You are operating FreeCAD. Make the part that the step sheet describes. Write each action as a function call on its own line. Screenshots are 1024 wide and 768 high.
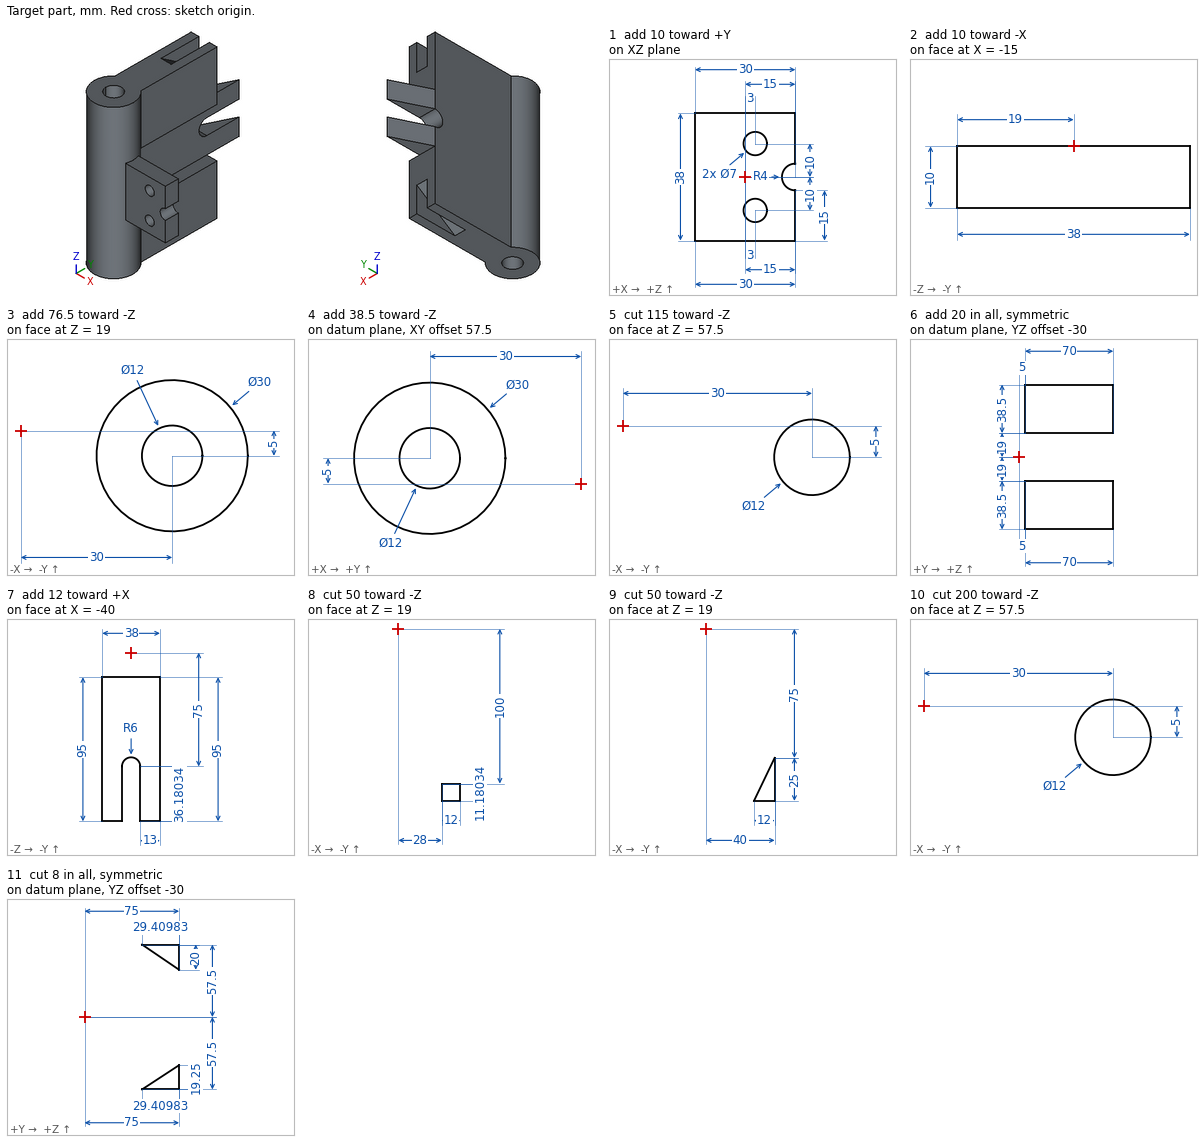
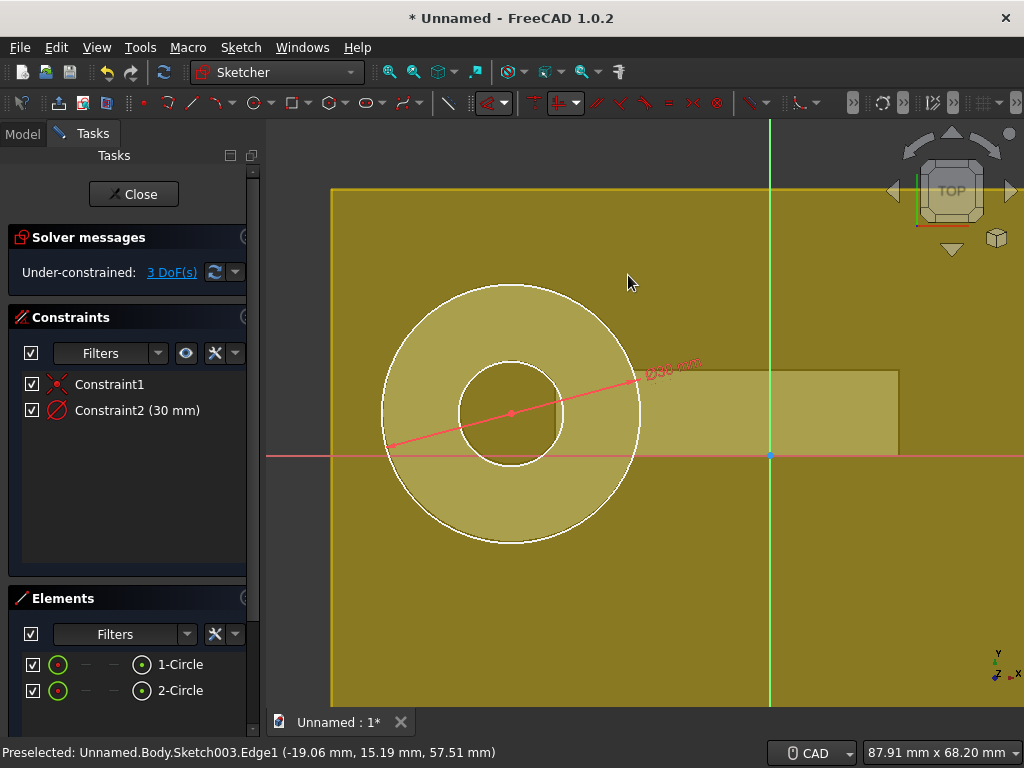
click(548, 377)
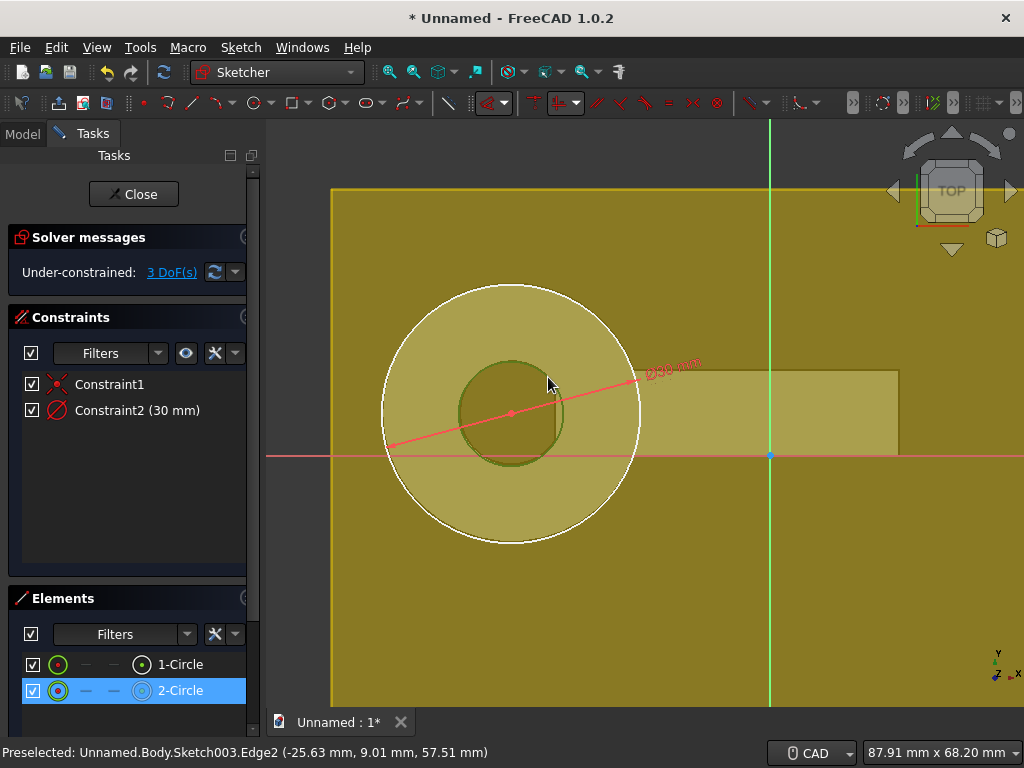
key(k)
key(o)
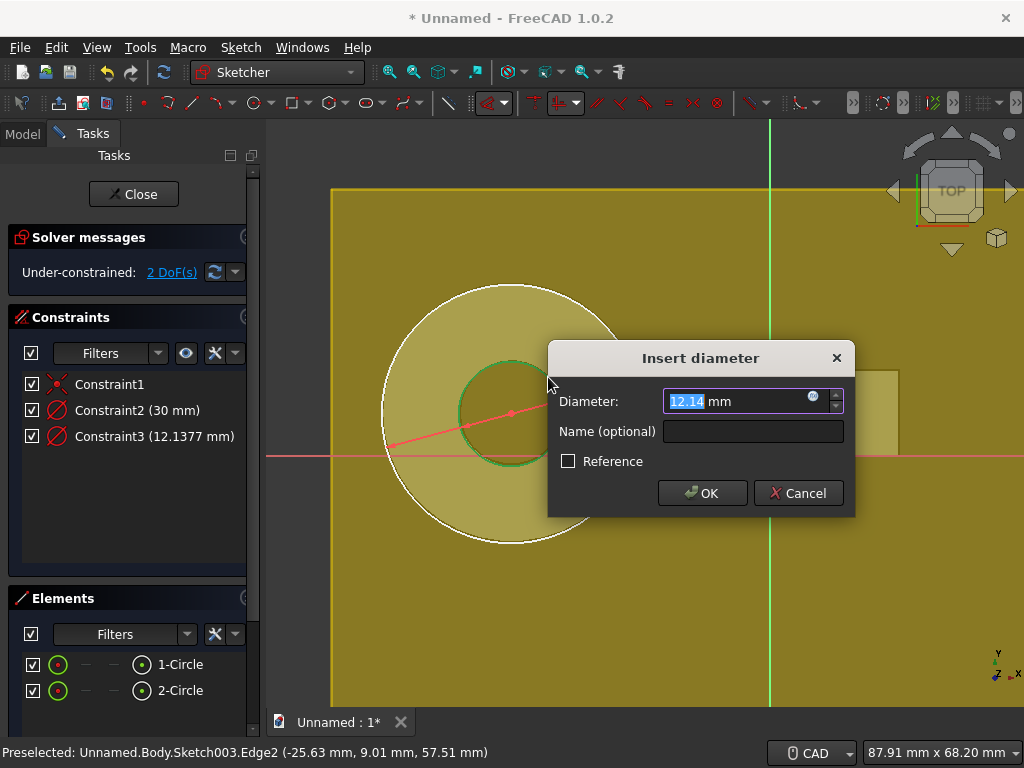
text(12)
key(Return)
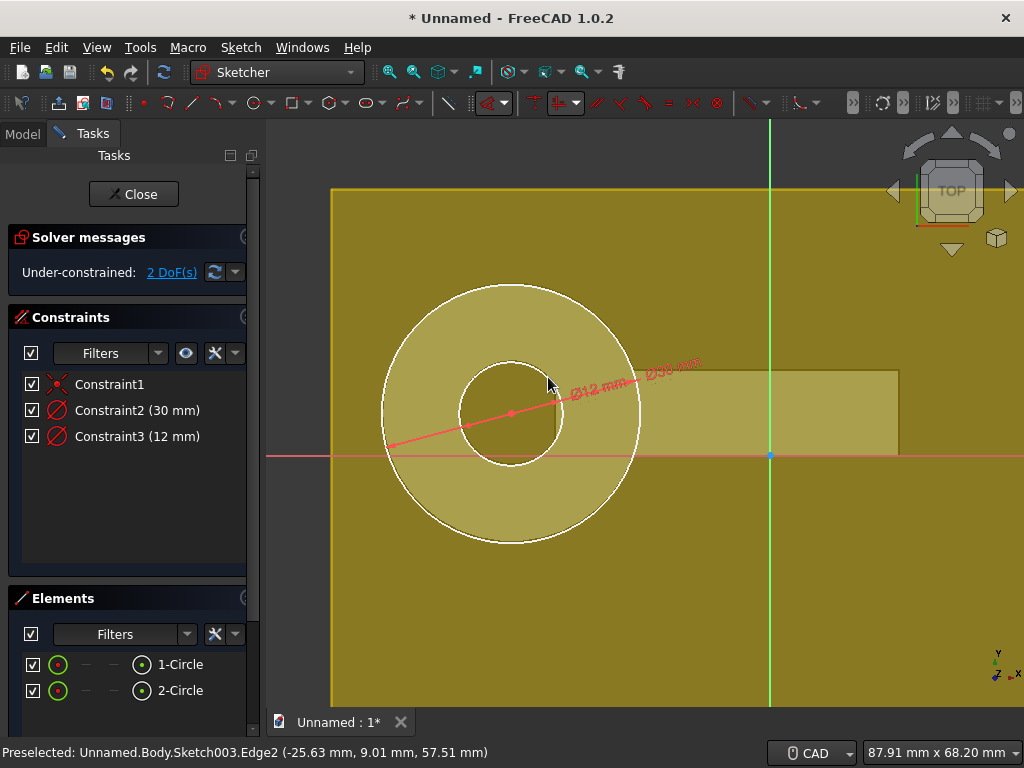
click(511, 414)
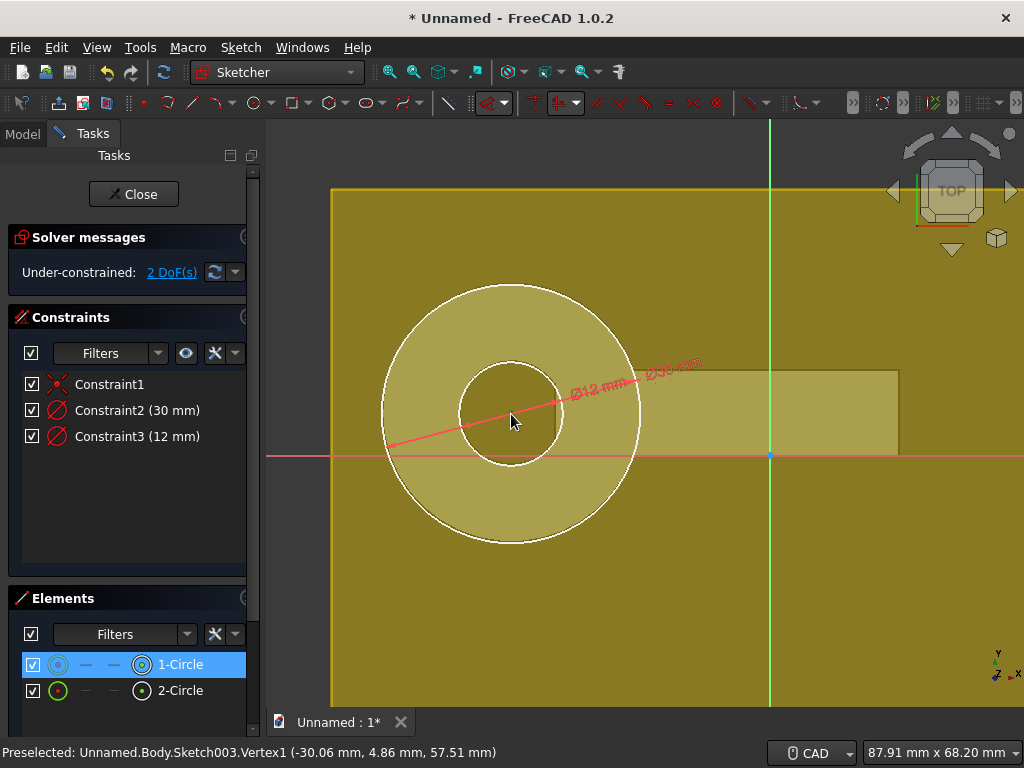
key(i)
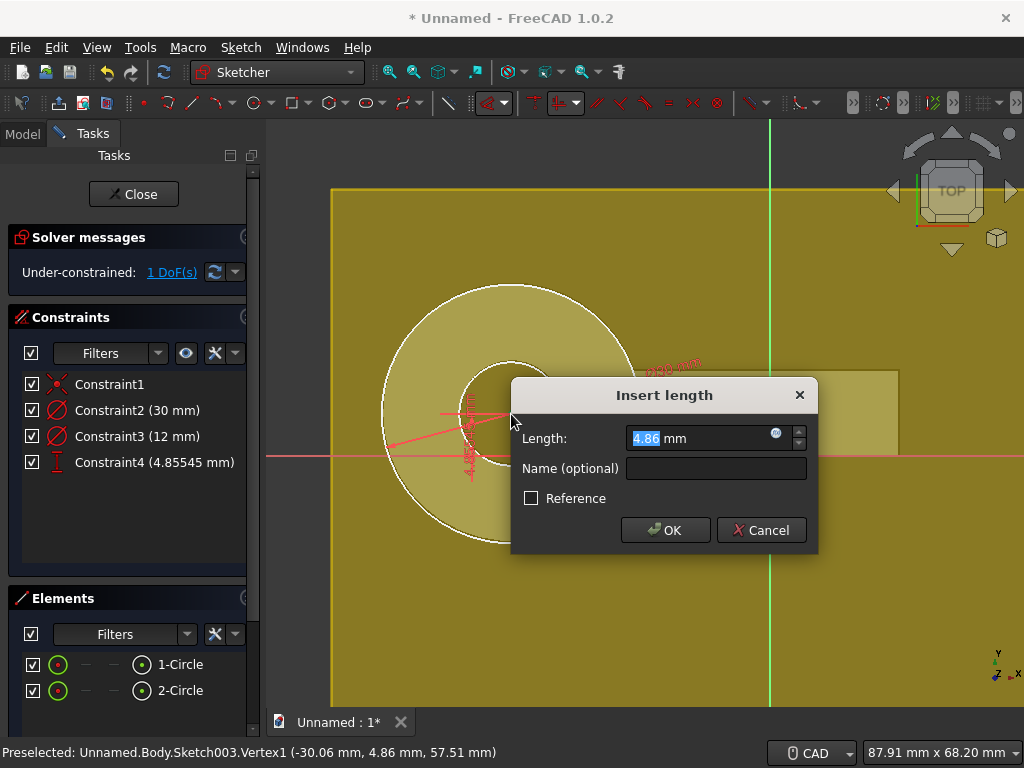
text(5)
key(Return)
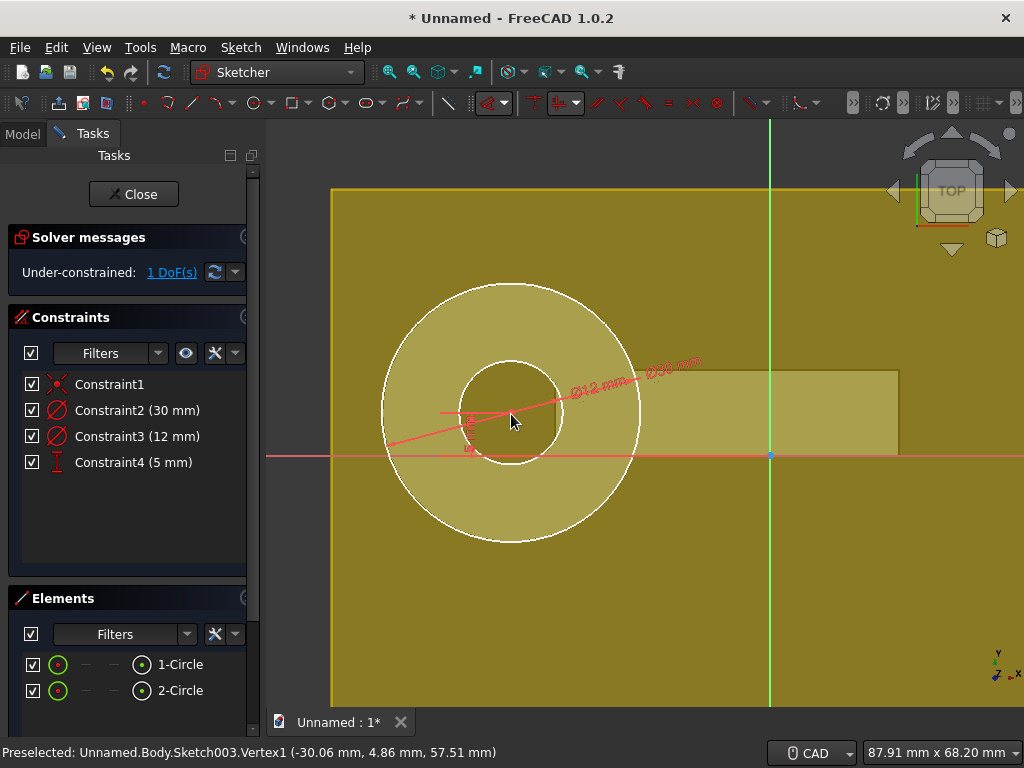
click(511, 413)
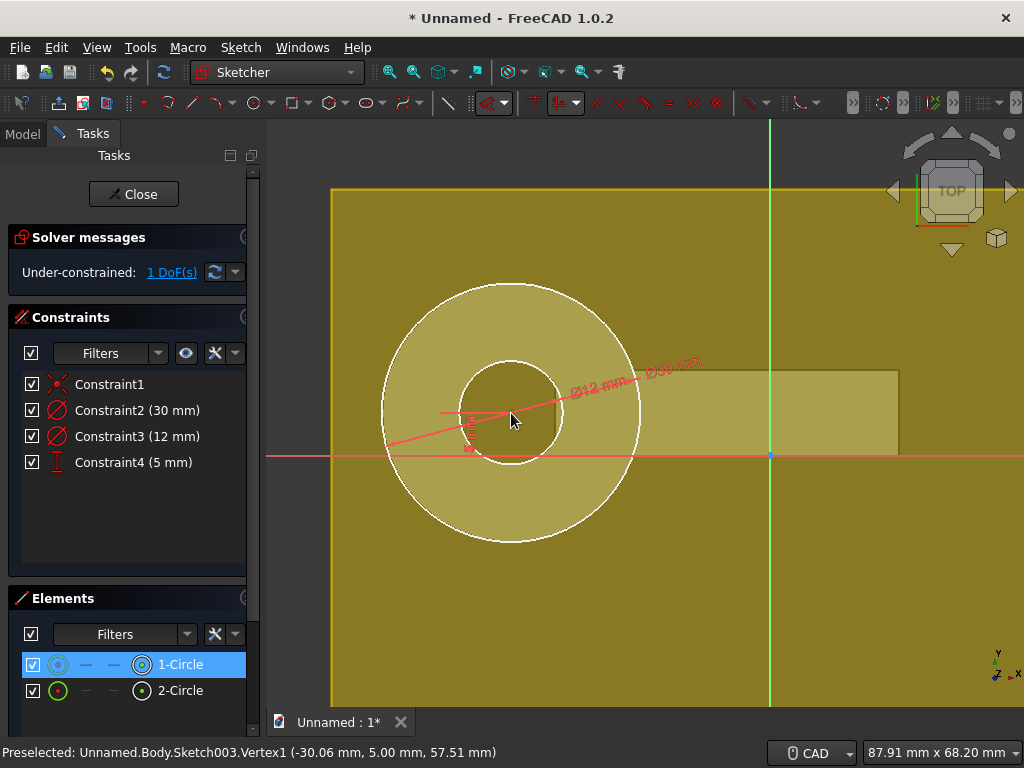
key(l)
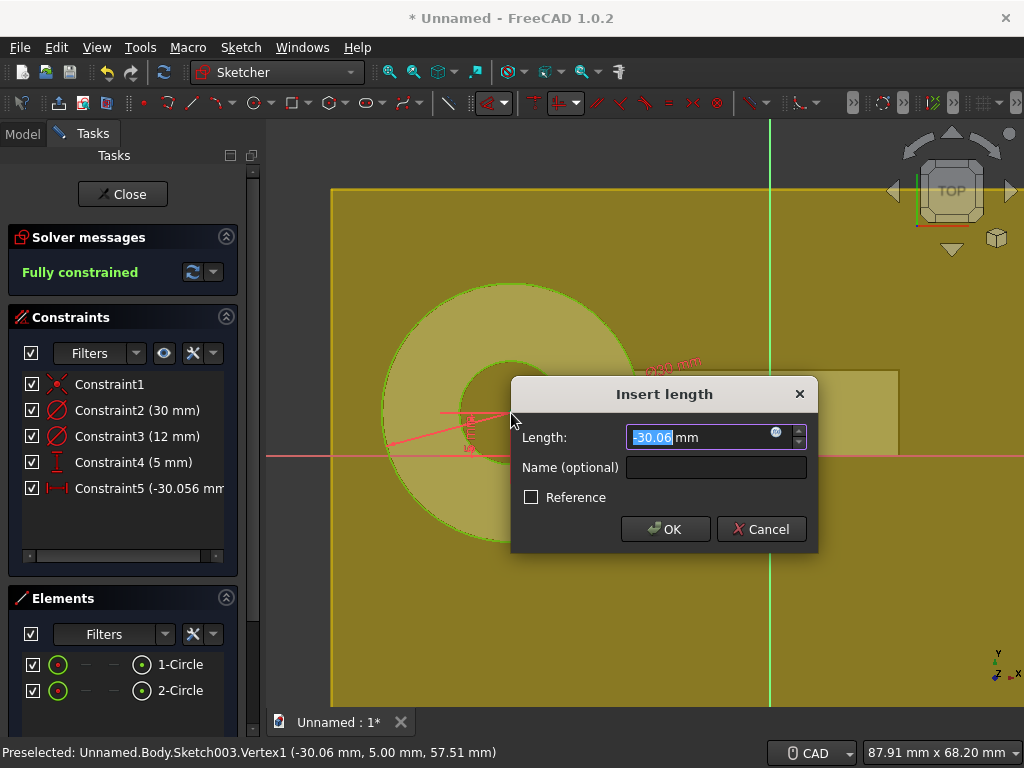
text(-30)
key(Return)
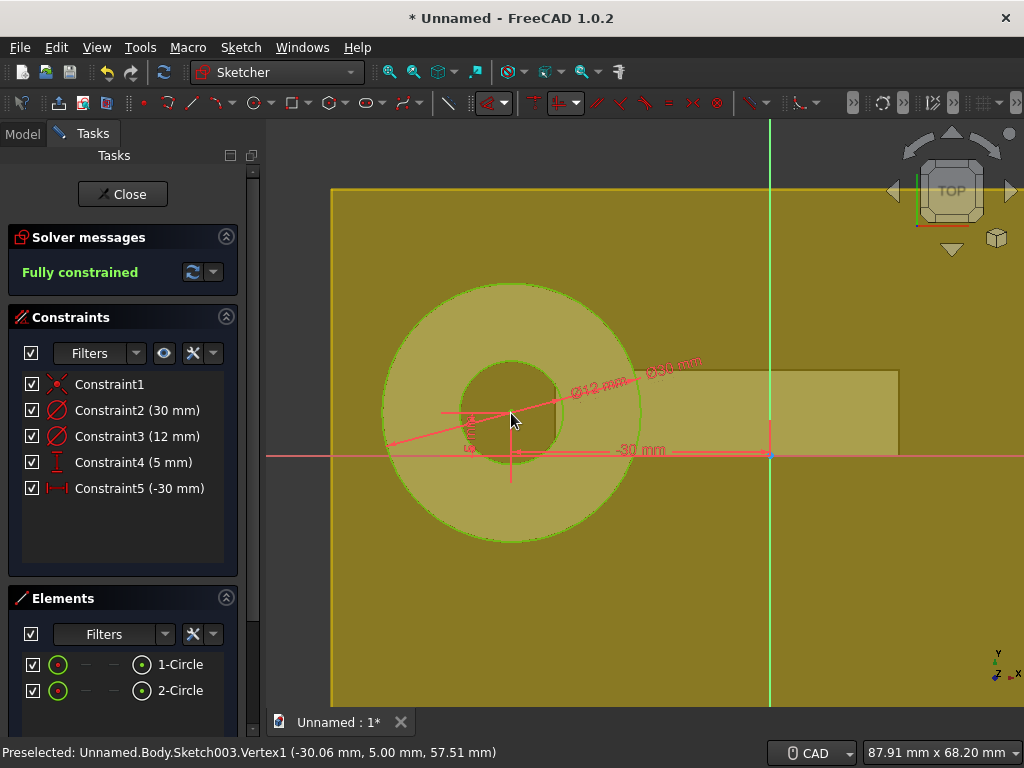
click(123, 194)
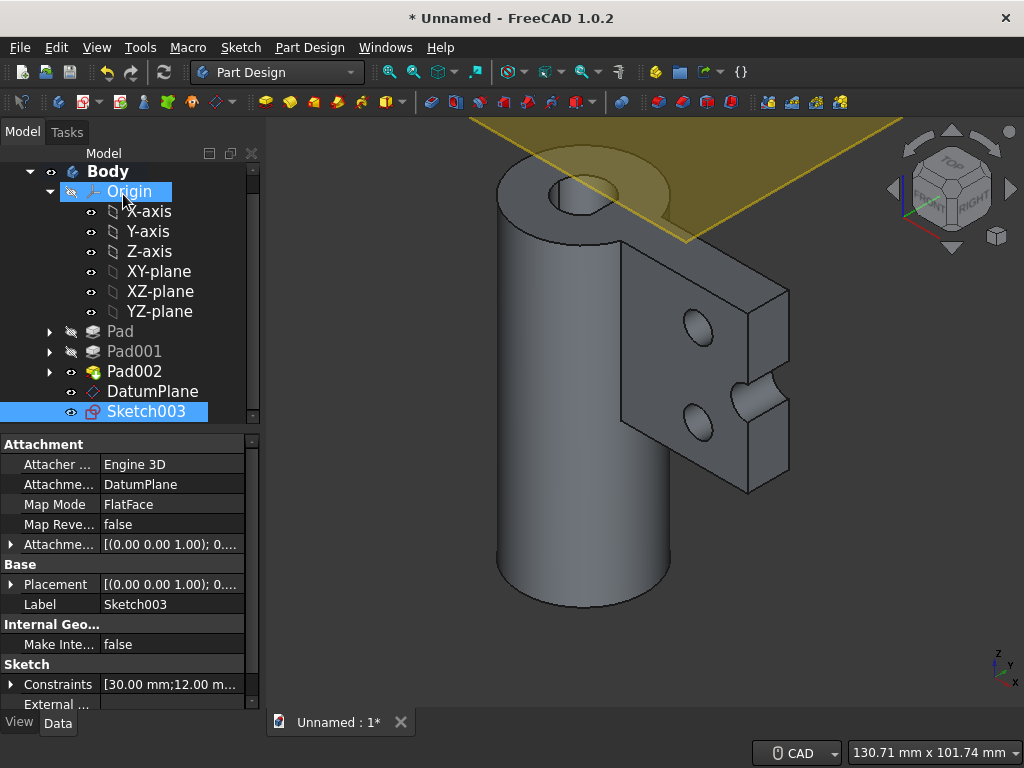
click(266, 102)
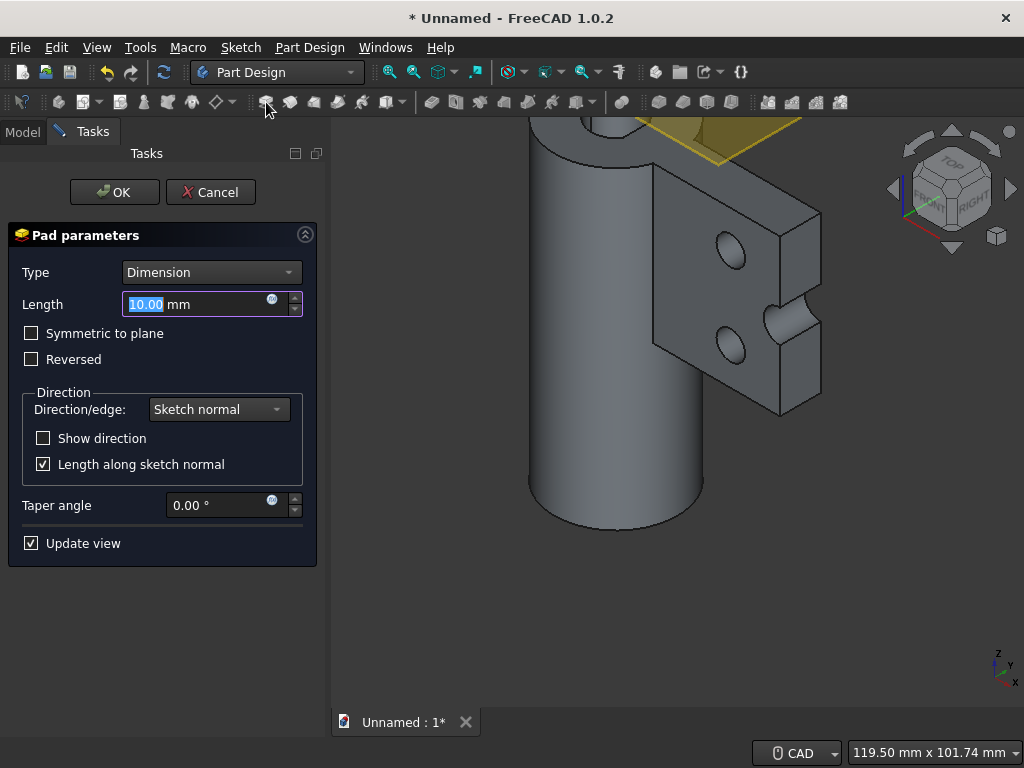
text(38.5)
key(Tab)